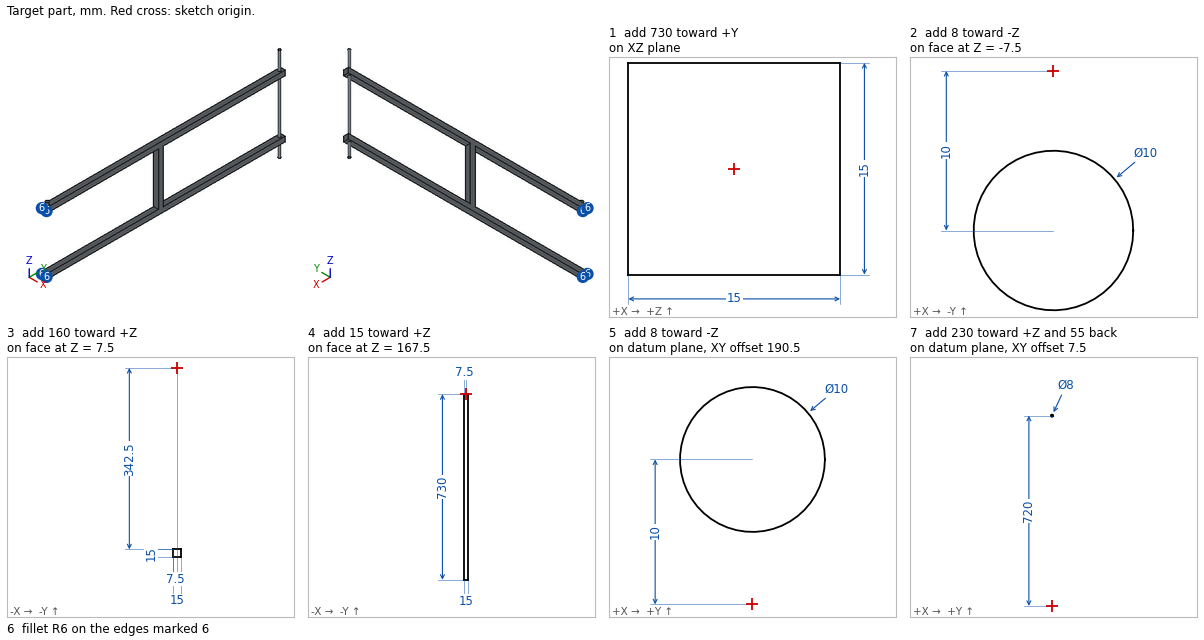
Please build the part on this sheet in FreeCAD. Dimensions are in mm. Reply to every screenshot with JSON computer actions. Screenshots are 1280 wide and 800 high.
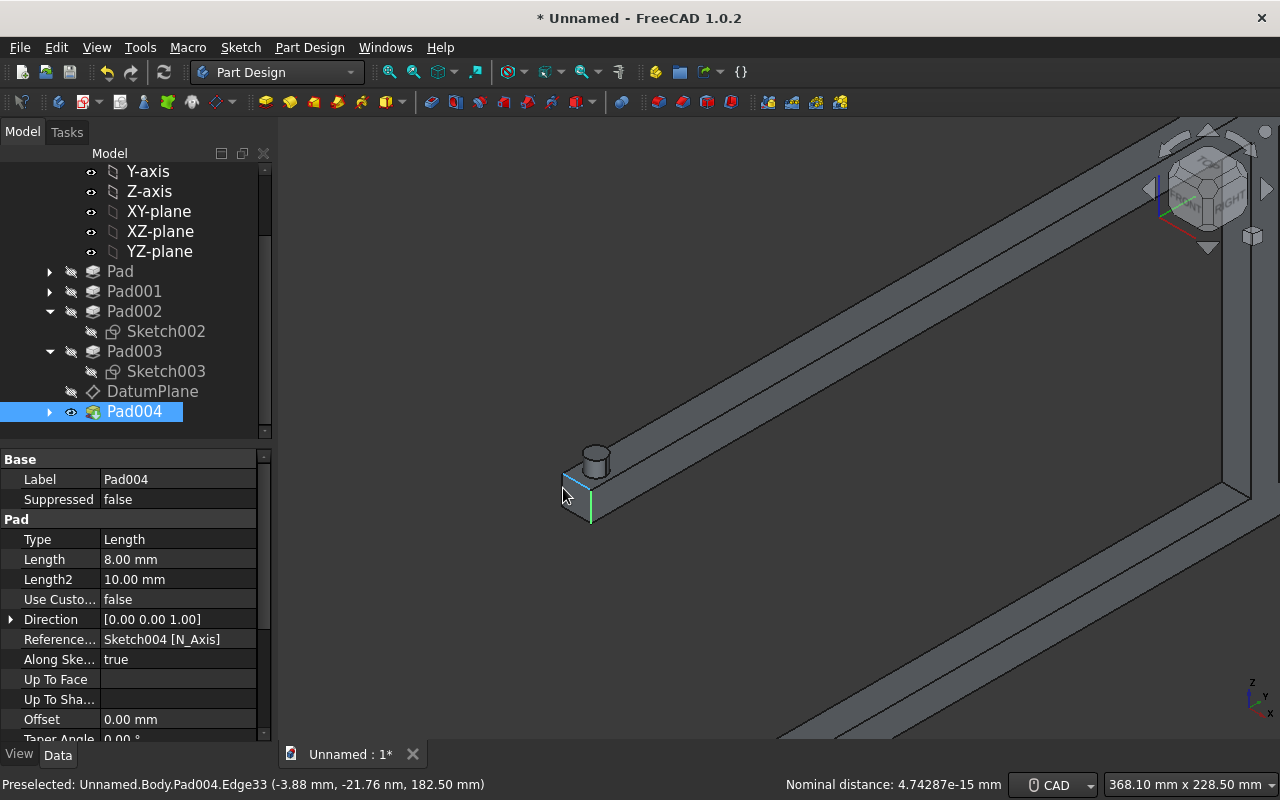
{"action": "left_click", "coordinate": [390, 72]}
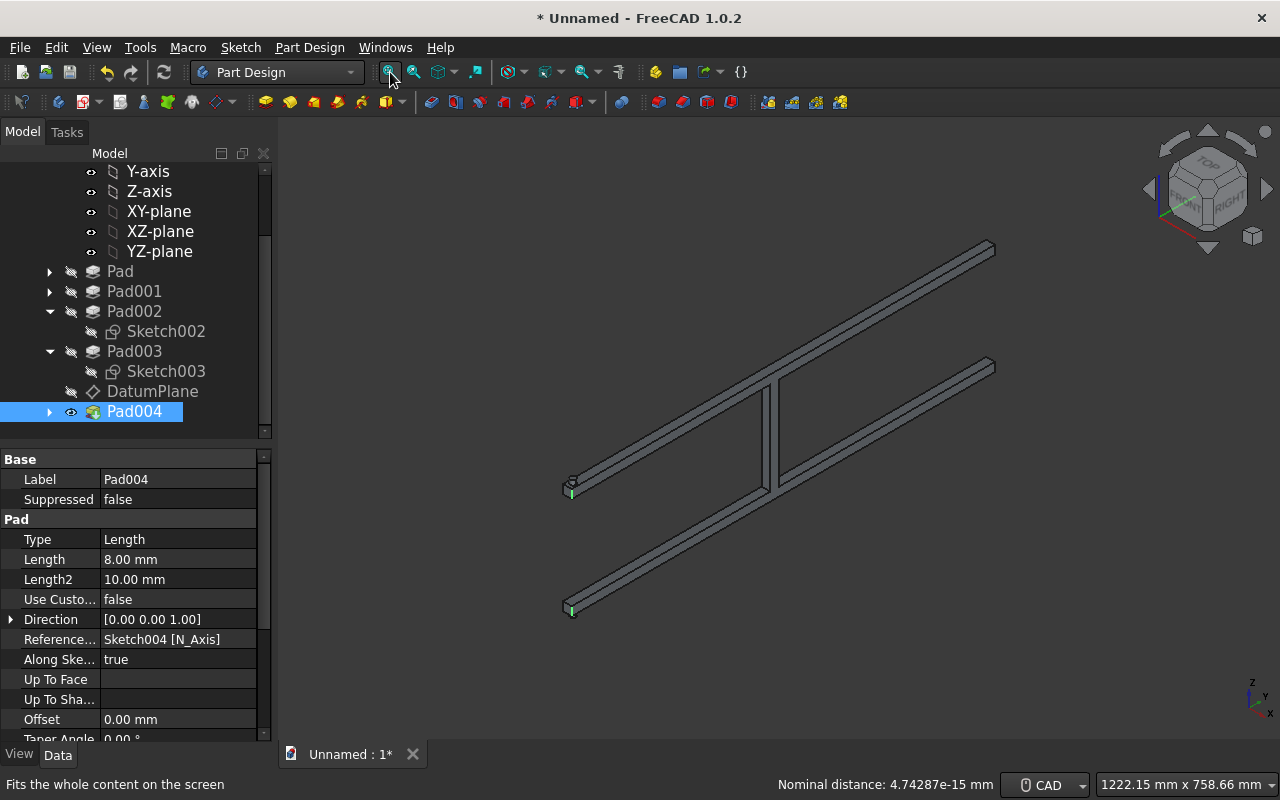
{"action": "key", "text": "1"}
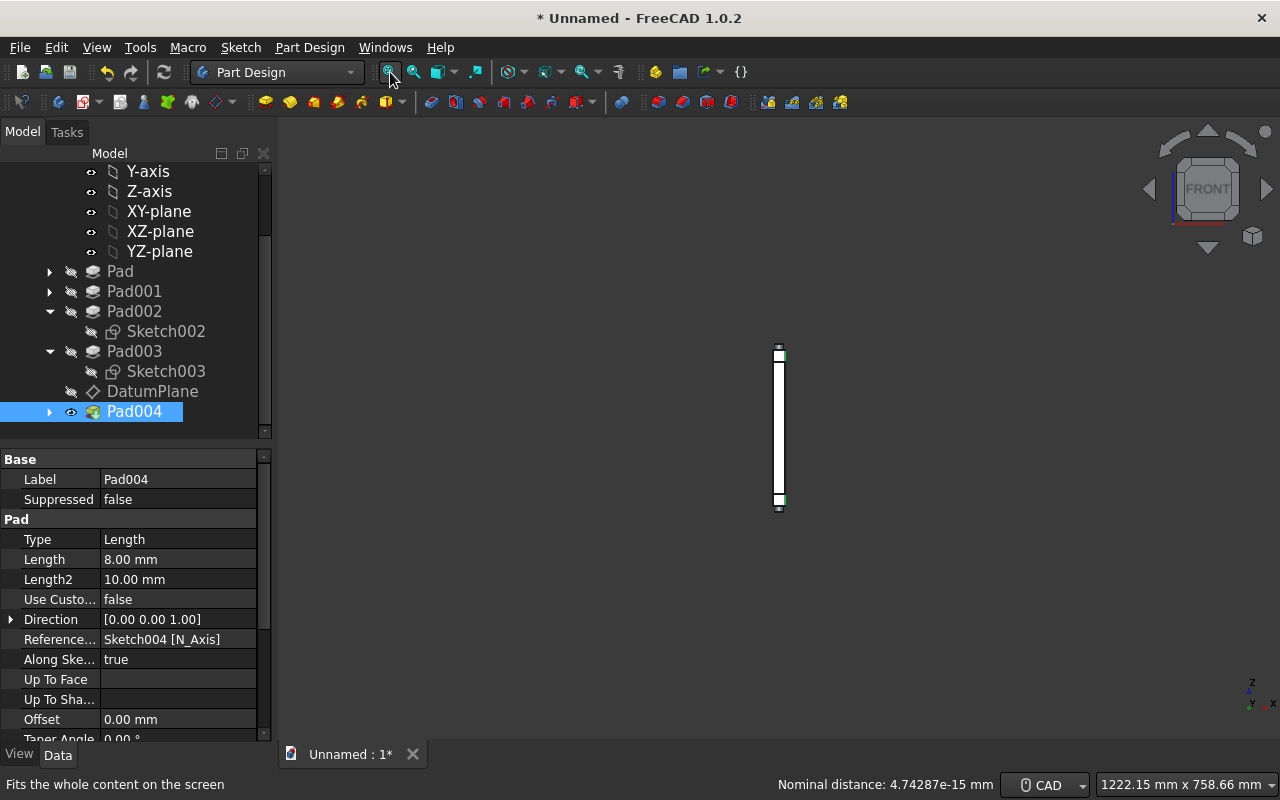
{"action": "left_click", "coordinate": [390, 72]}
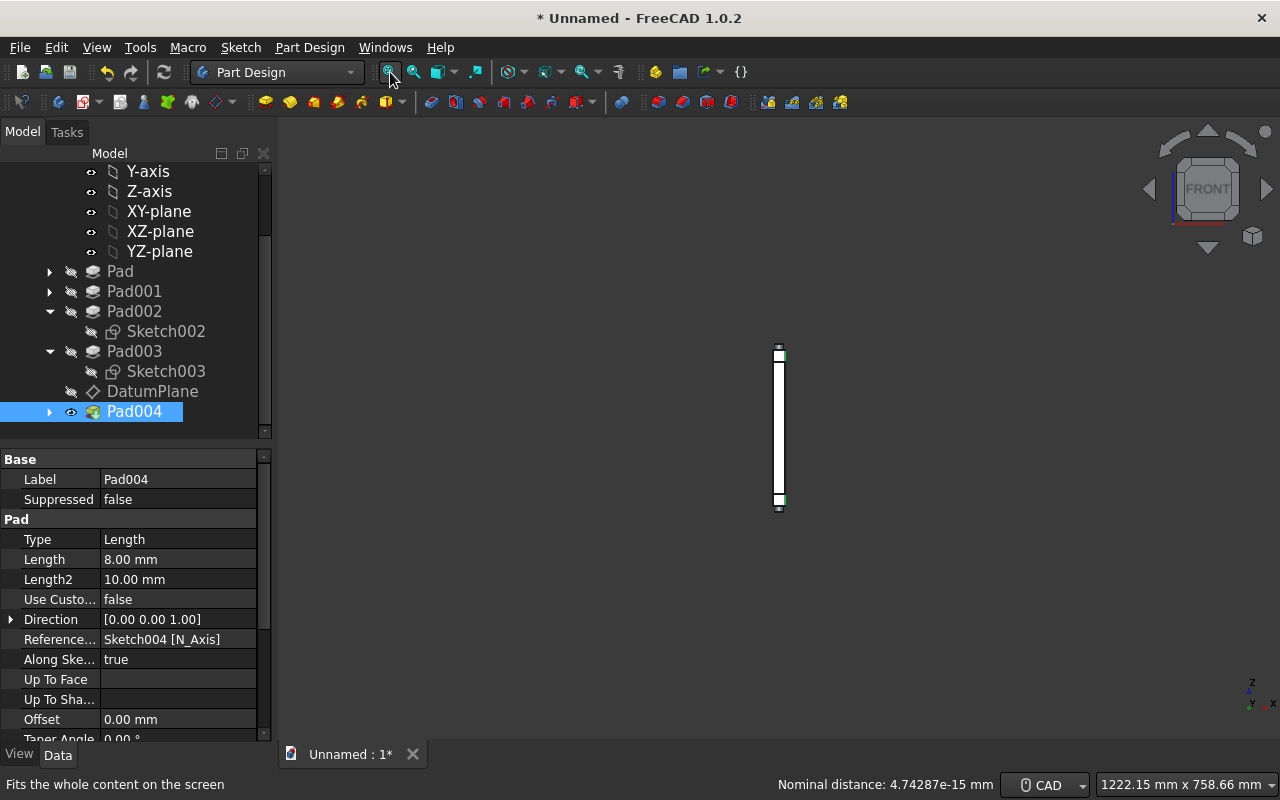
{"action": "left_click", "coordinate": [773, 359], "text": "ctrl"}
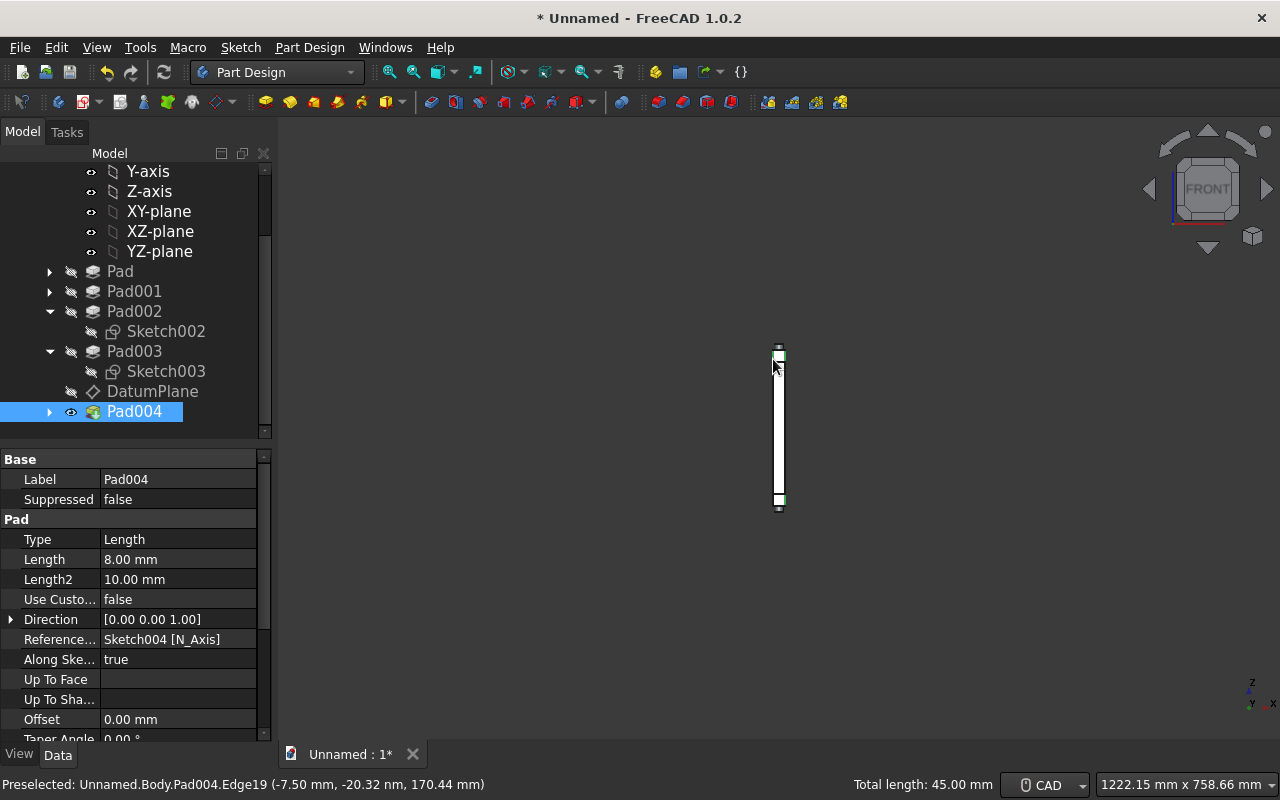
{"action": "scroll", "coordinate": [773, 499], "scroll_direction": "up", "scroll_amount": 6}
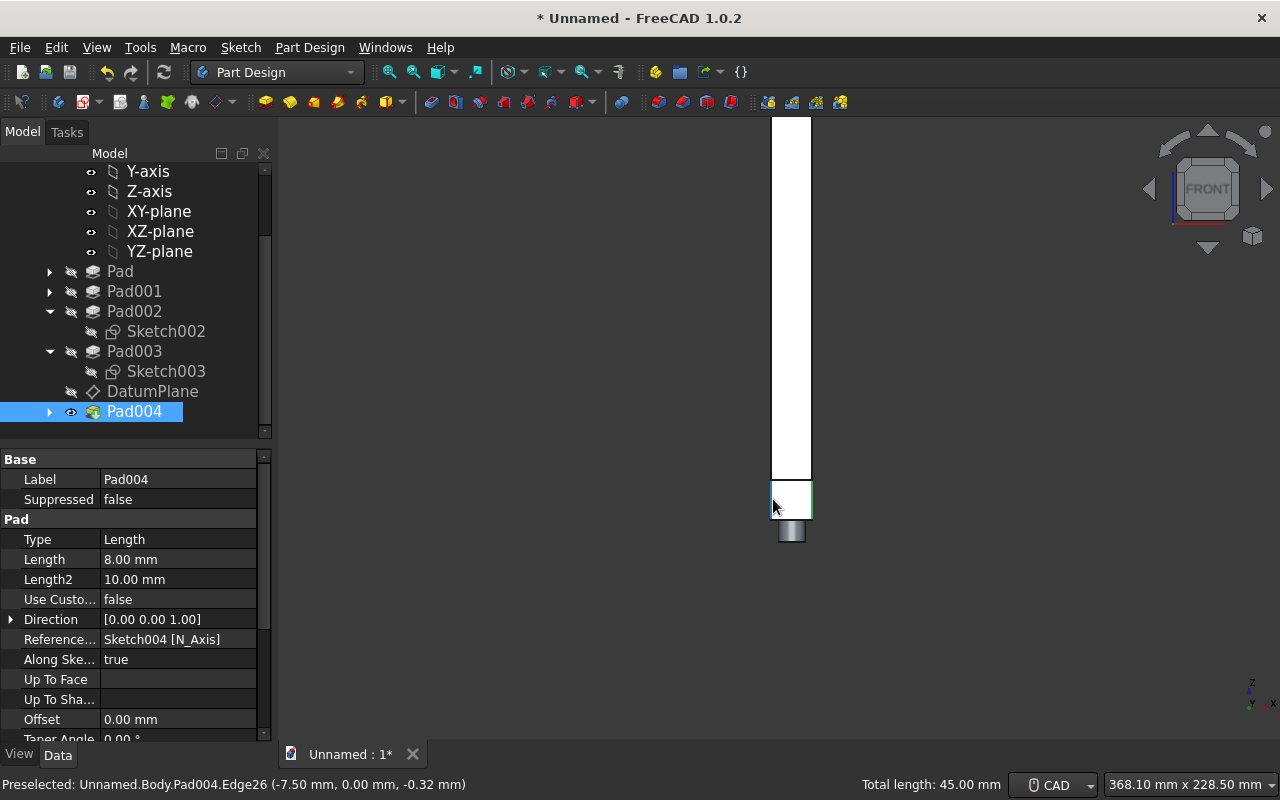
{"action": "left_click", "coordinate": [390, 72]}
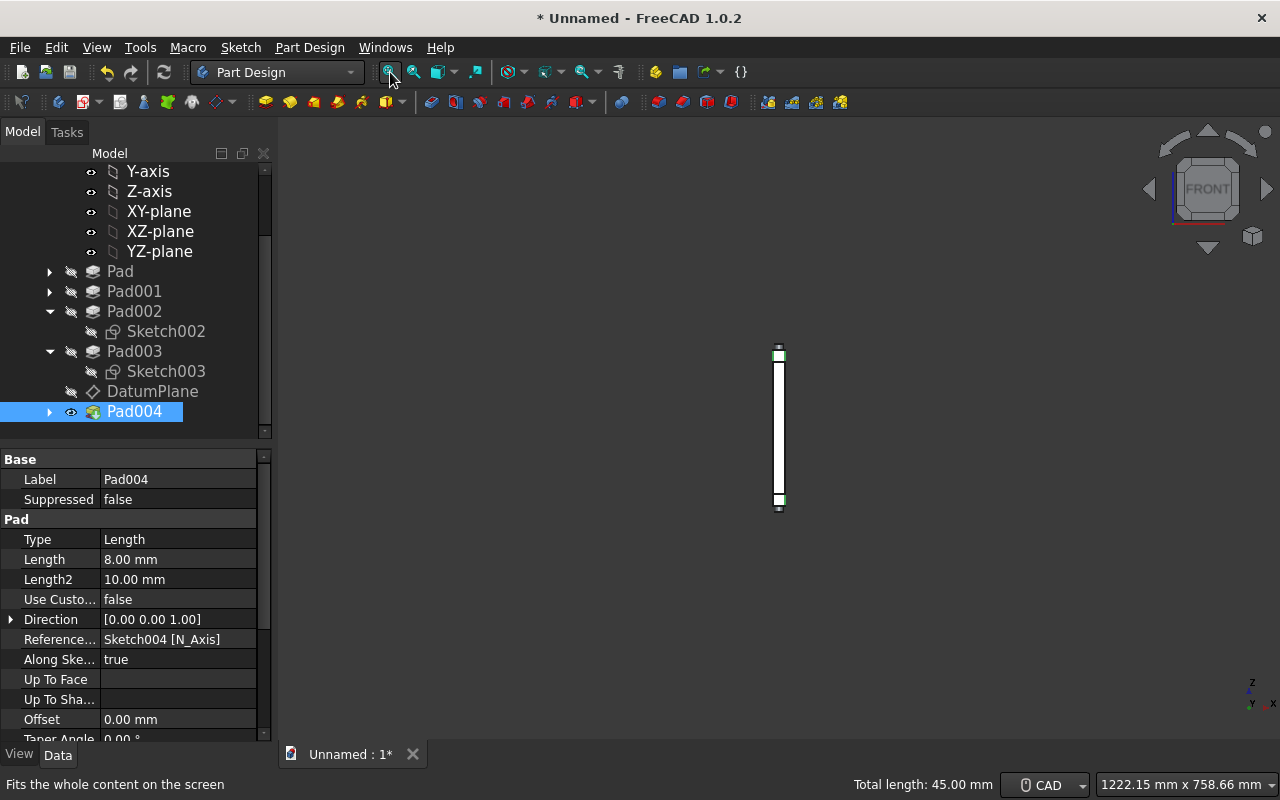
{"action": "key", "text": "3"}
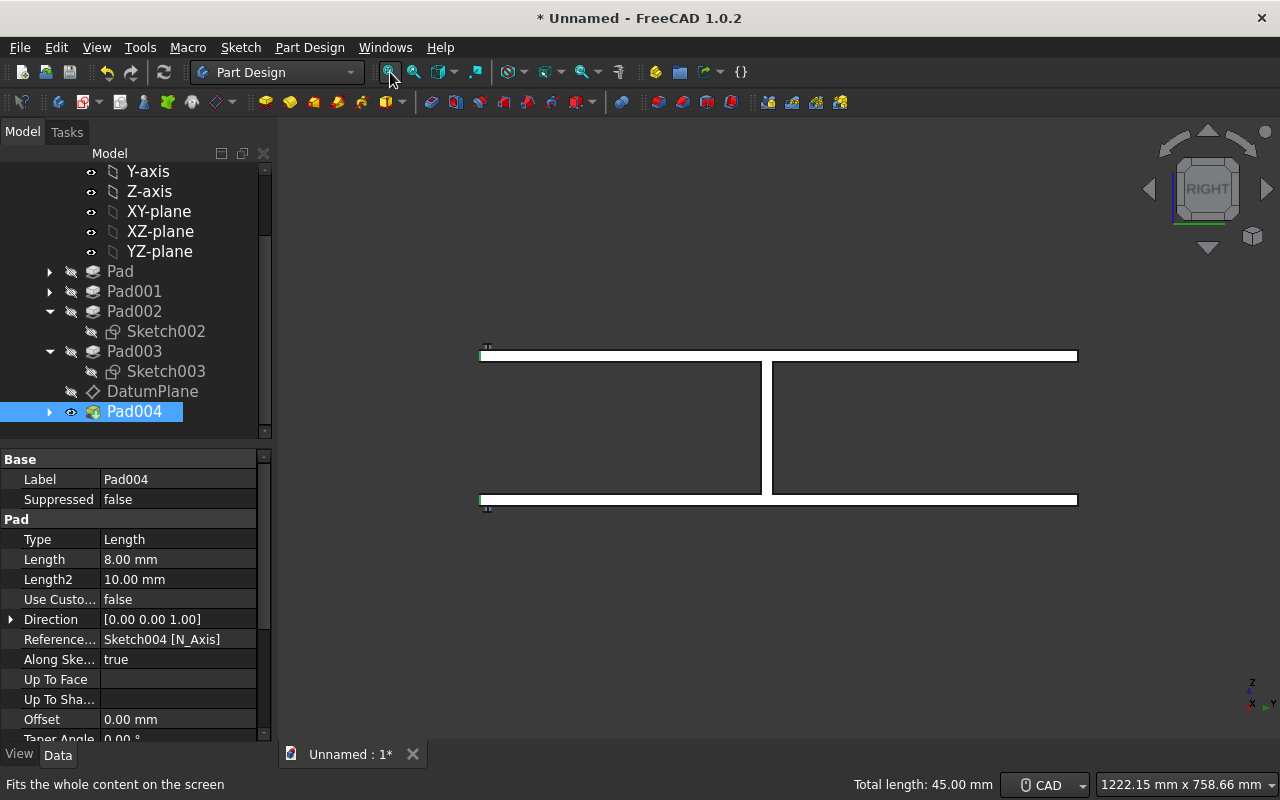
{"action": "scroll", "coordinate": [480, 499], "scroll_direction": "up", "scroll_amount": 6}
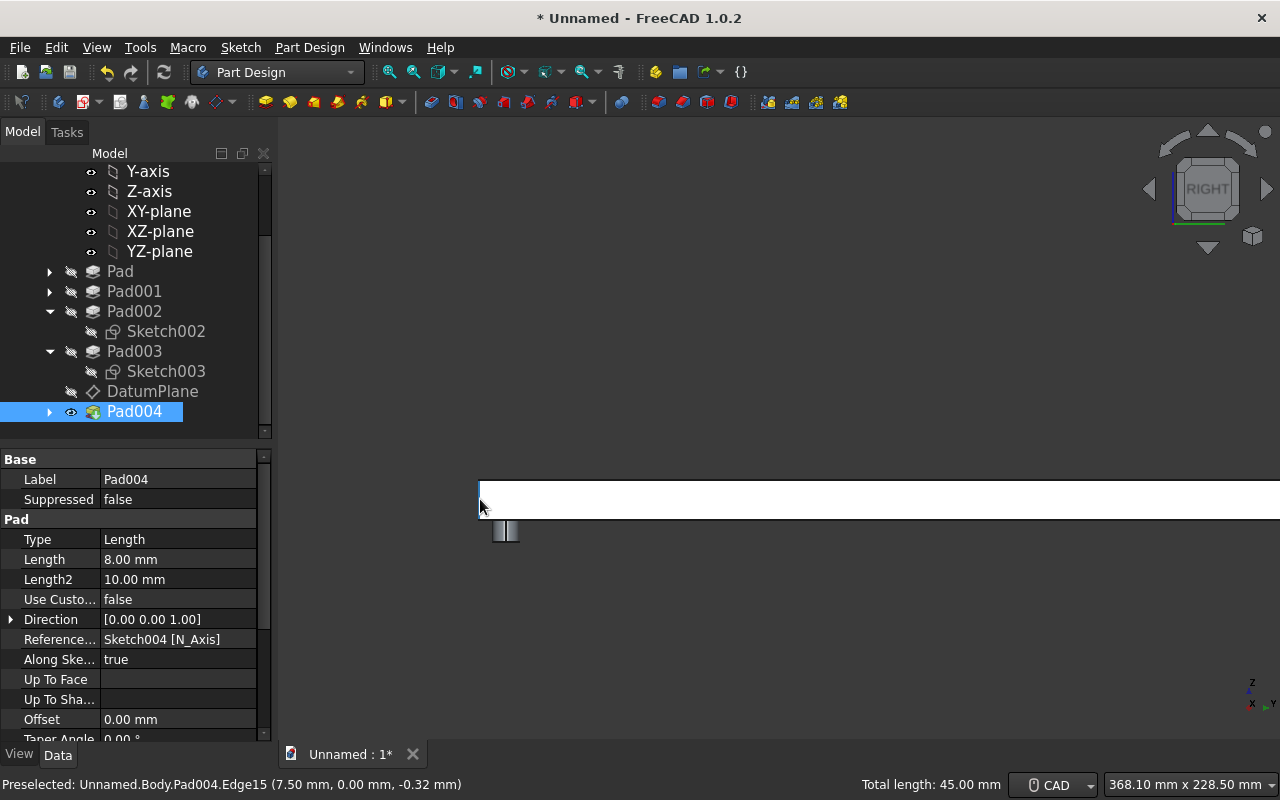
{"action": "left_click", "coordinate": [390, 72]}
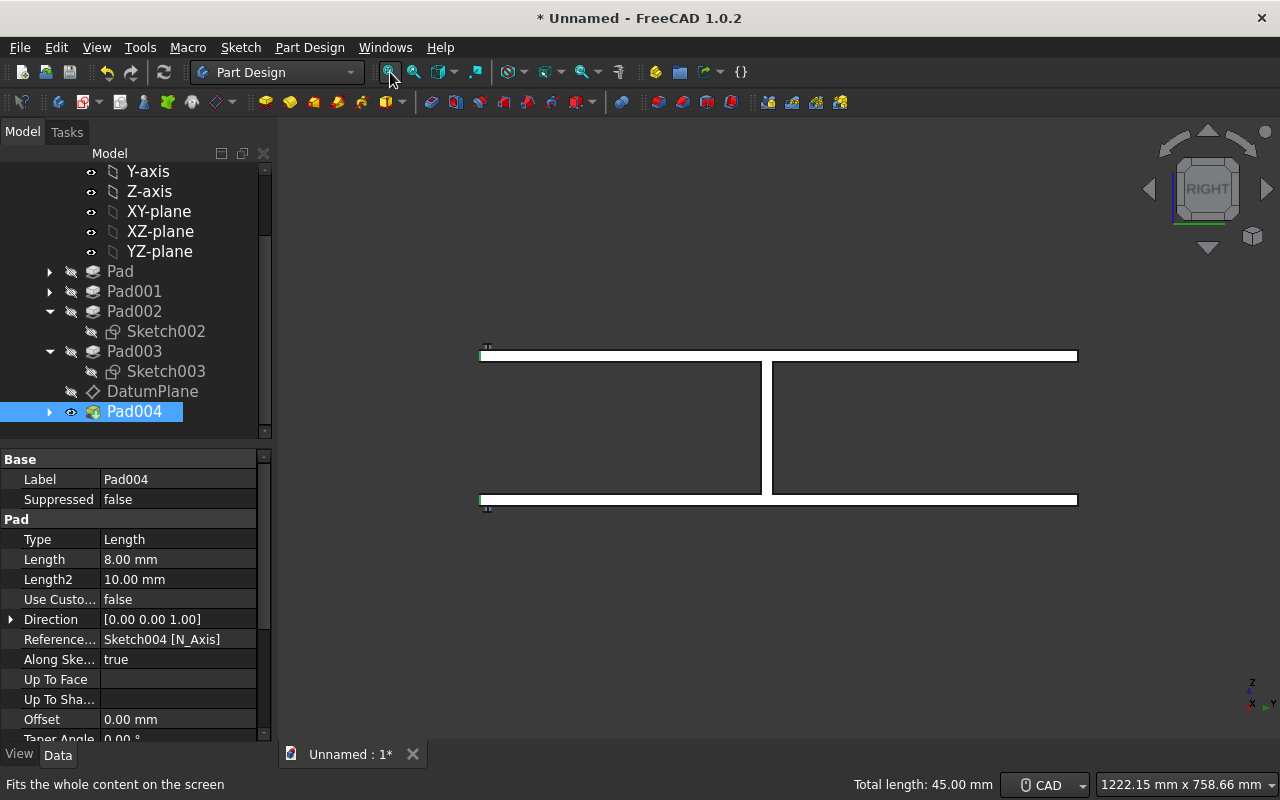
{"action": "key", "text": "5"}